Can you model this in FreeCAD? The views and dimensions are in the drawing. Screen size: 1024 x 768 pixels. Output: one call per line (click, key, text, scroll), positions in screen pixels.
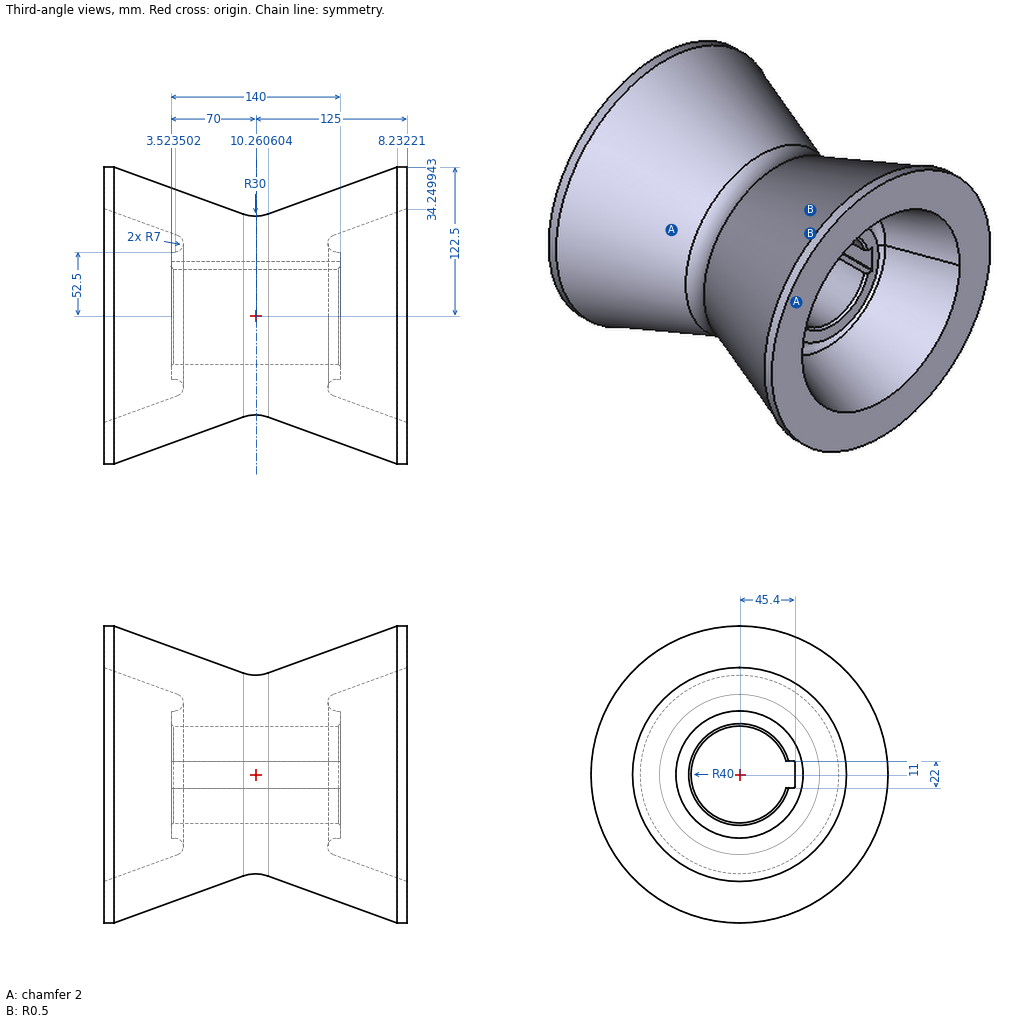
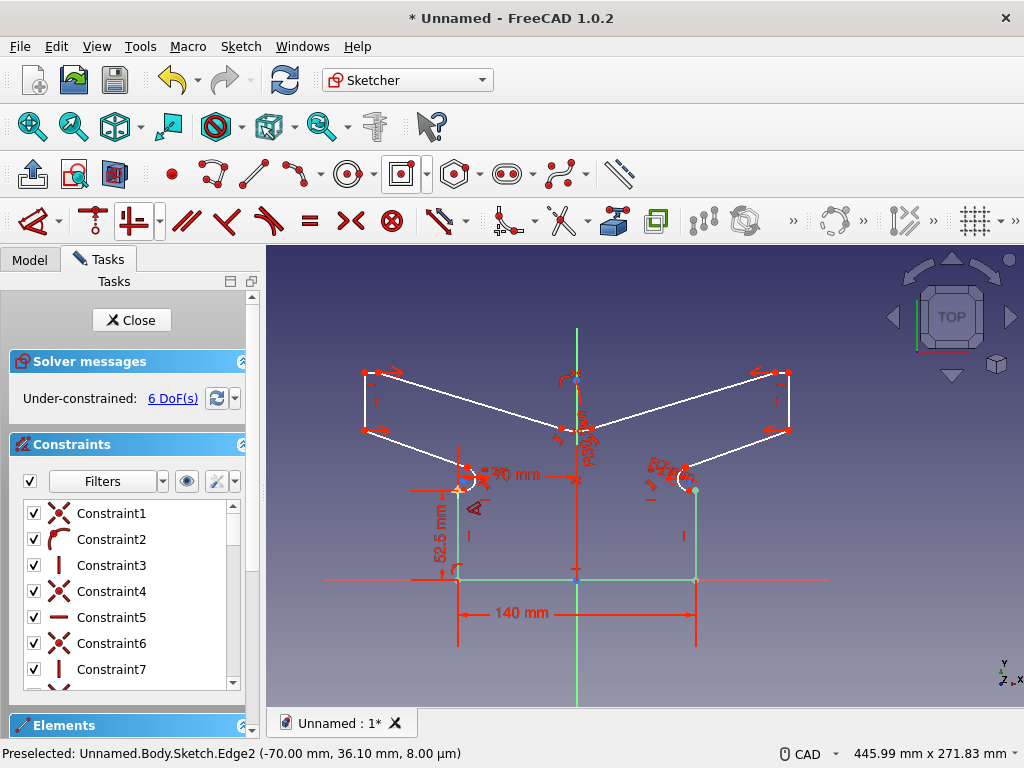
click(789, 431)
click(683, 614)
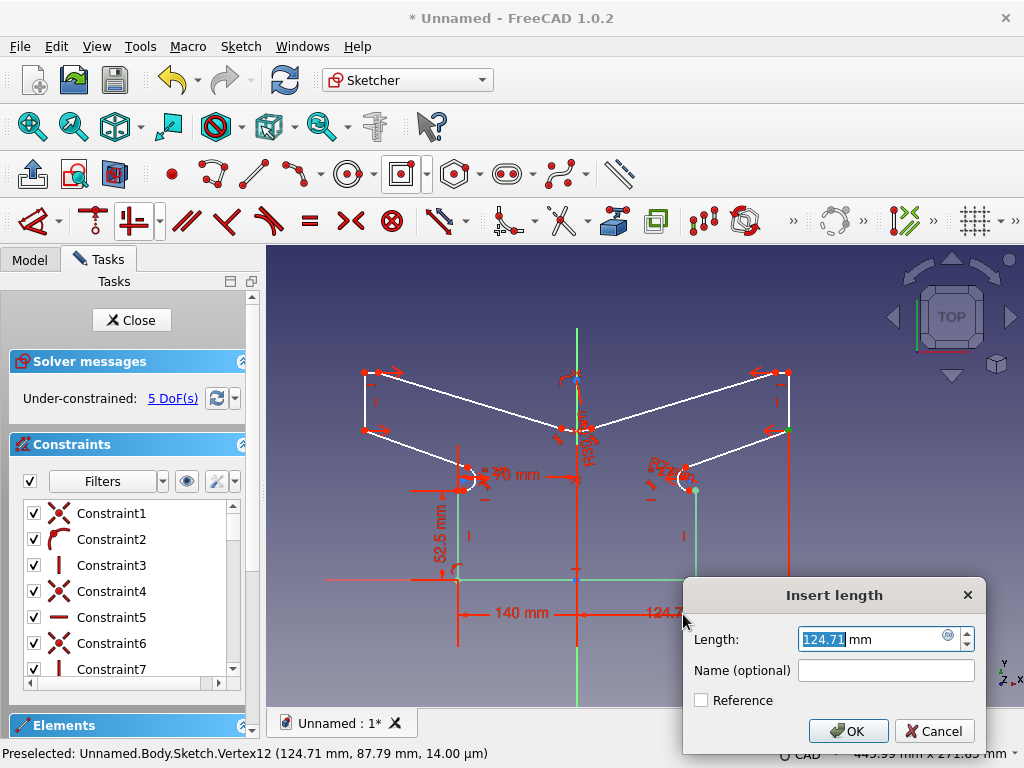
text(125)
key(Return)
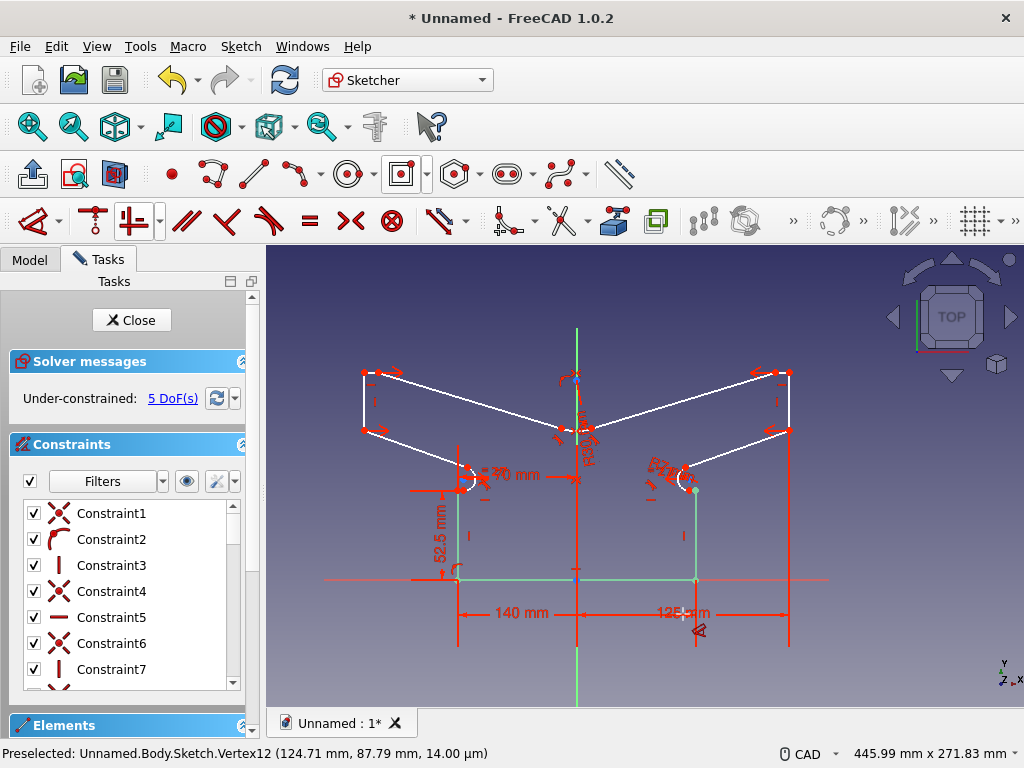
click(789, 373)
click(823, 477)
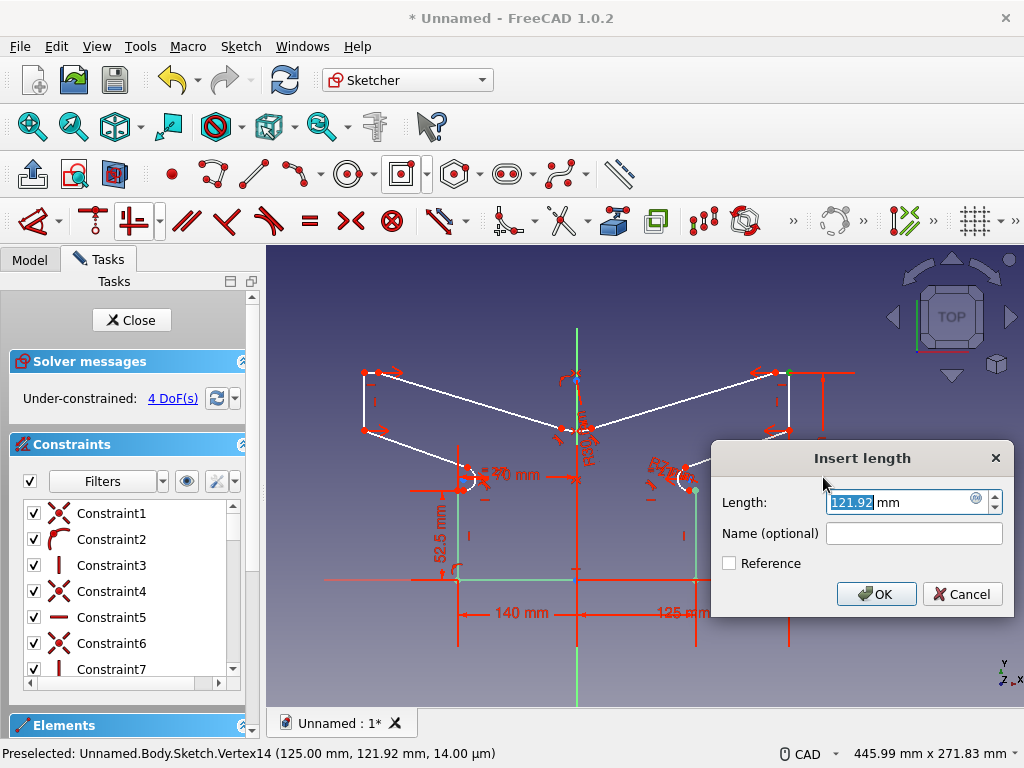
text(122.5)
key(Return)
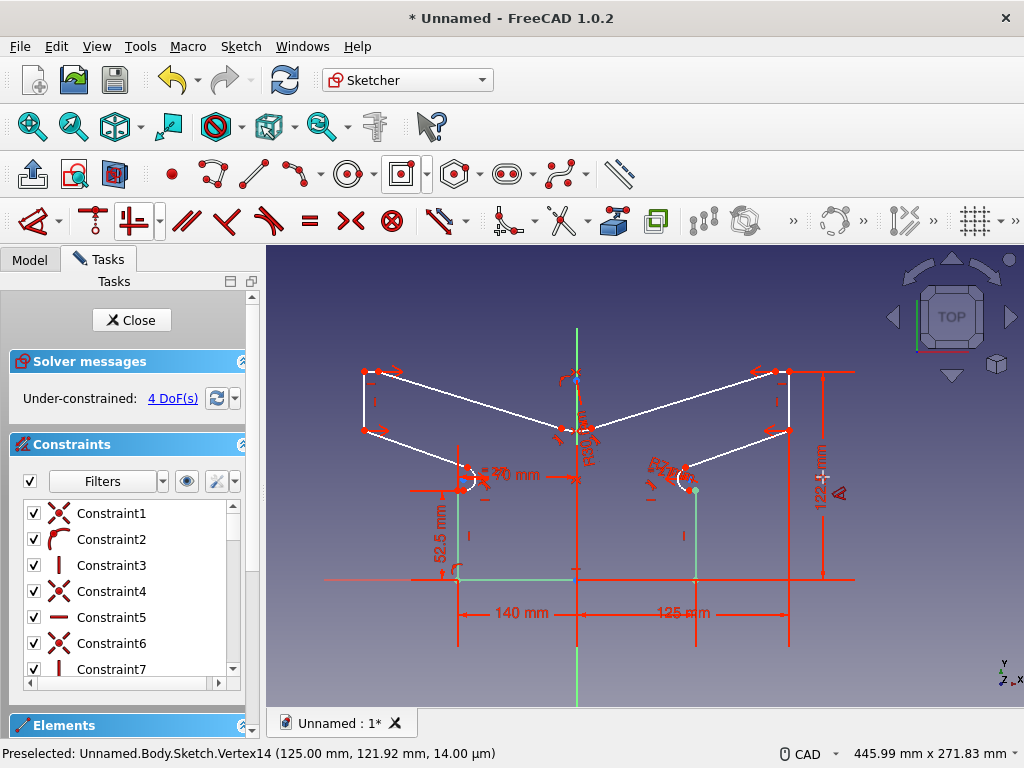
scroll(782, 372, up, 6)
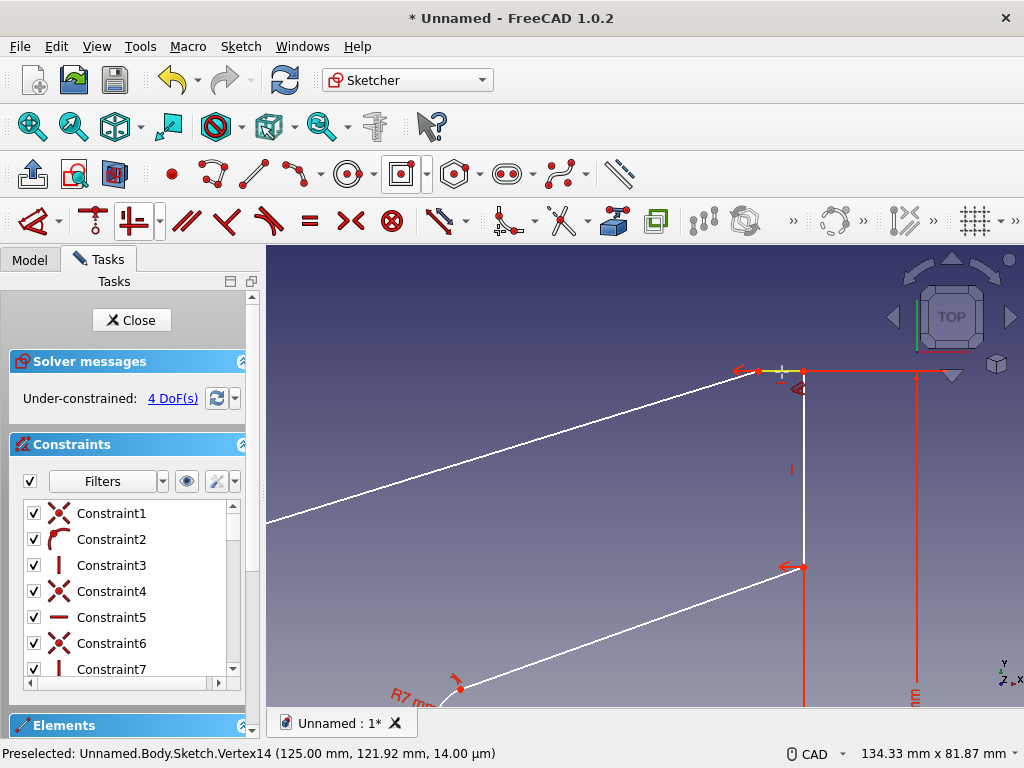
click(781, 371)
click(781, 337)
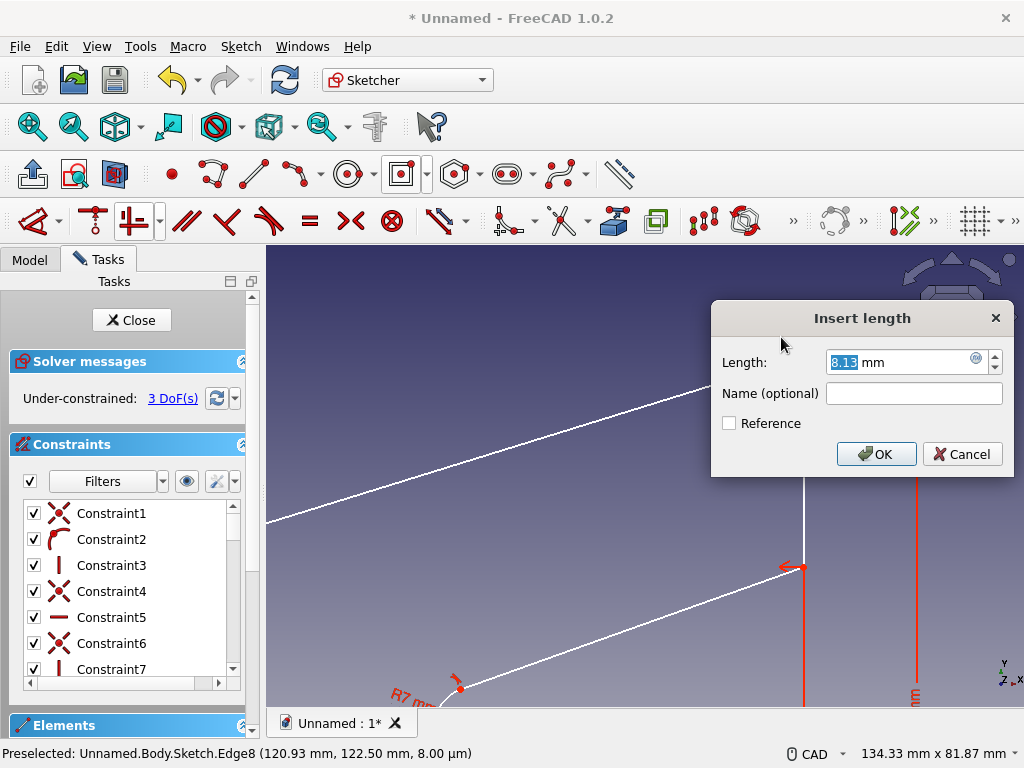
text(8.23221)
key(Return)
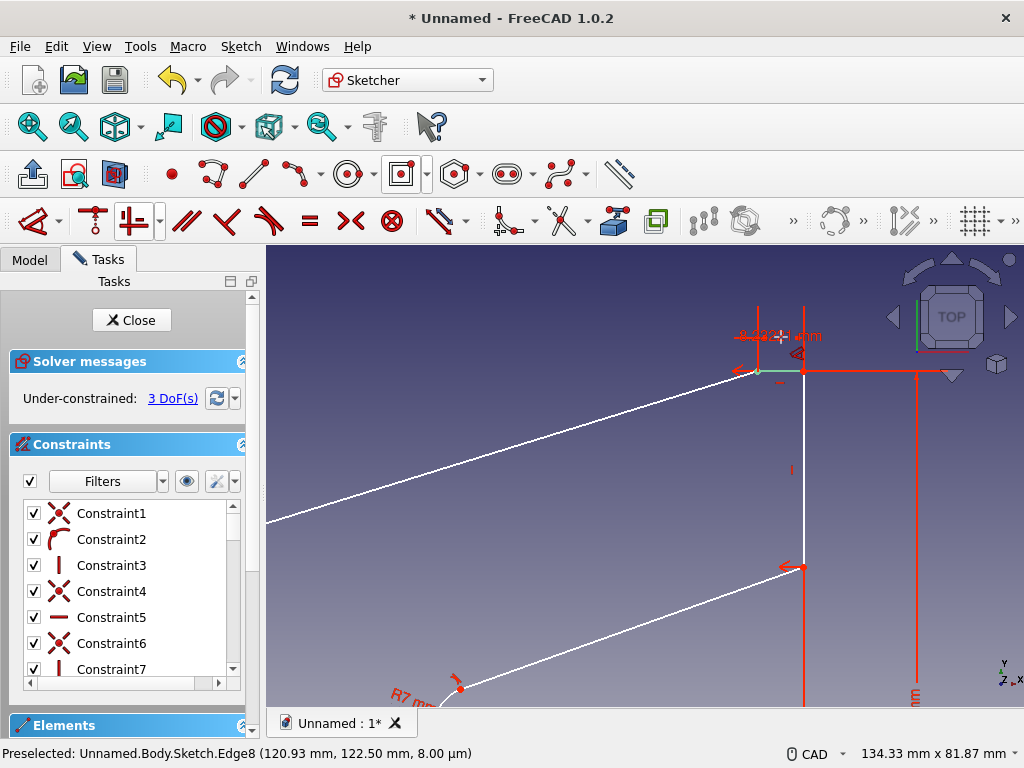
scroll(782, 372, down, 6)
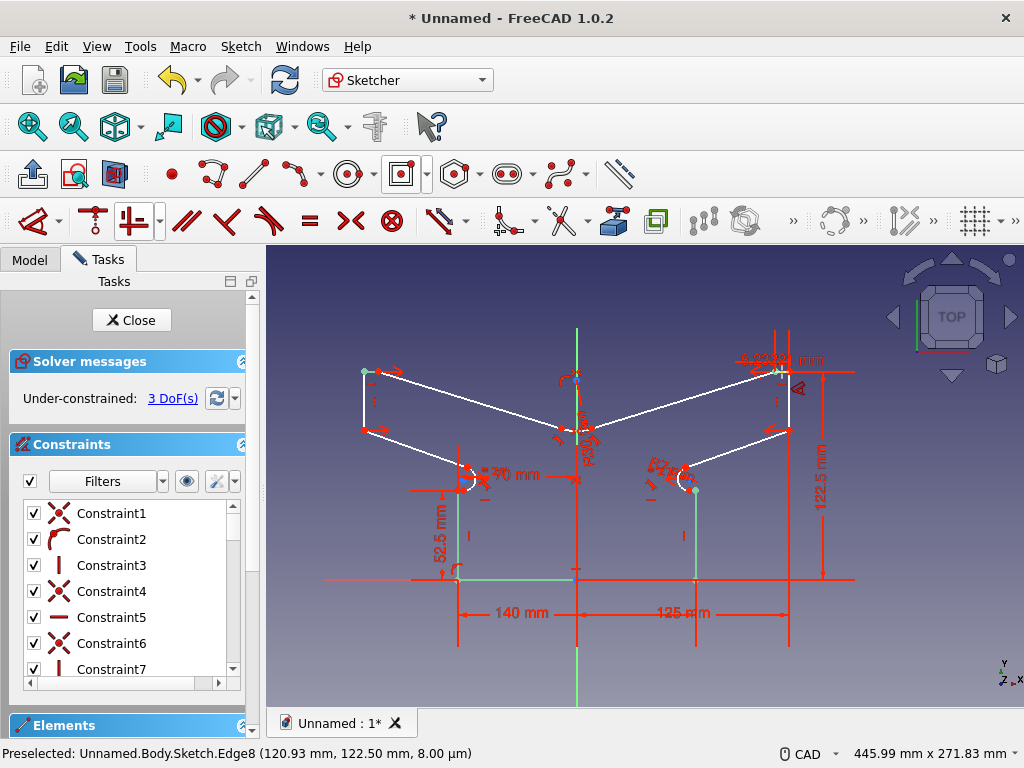
scroll(461, 491, up, 10)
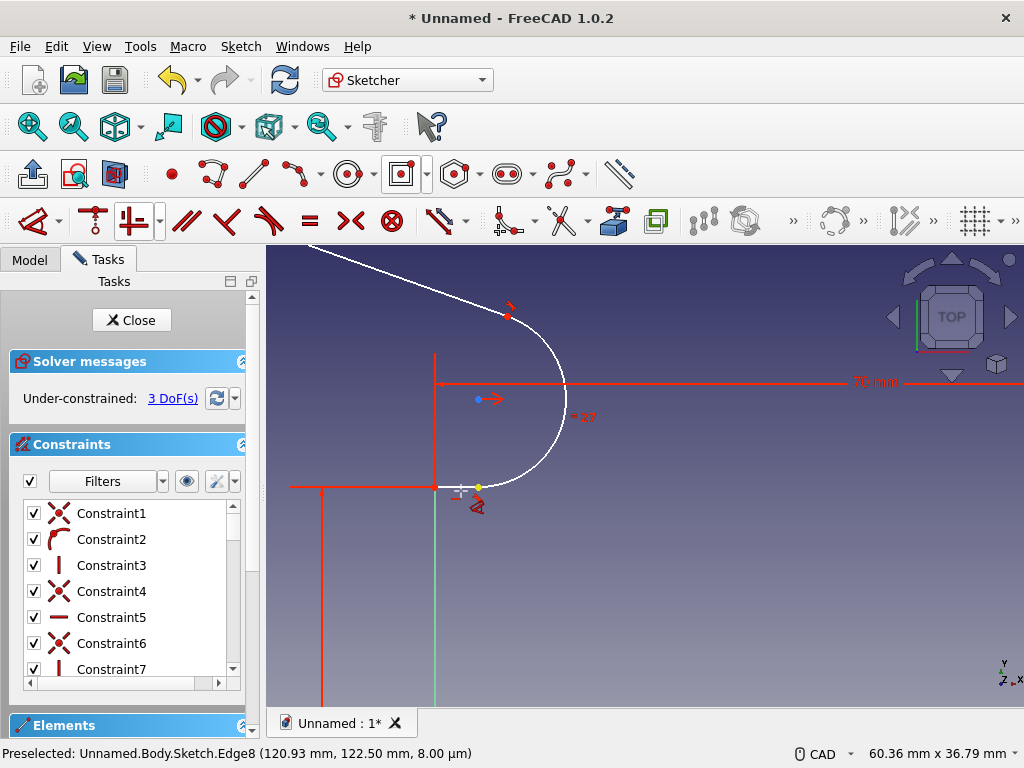
click(456, 487)
click(456, 521)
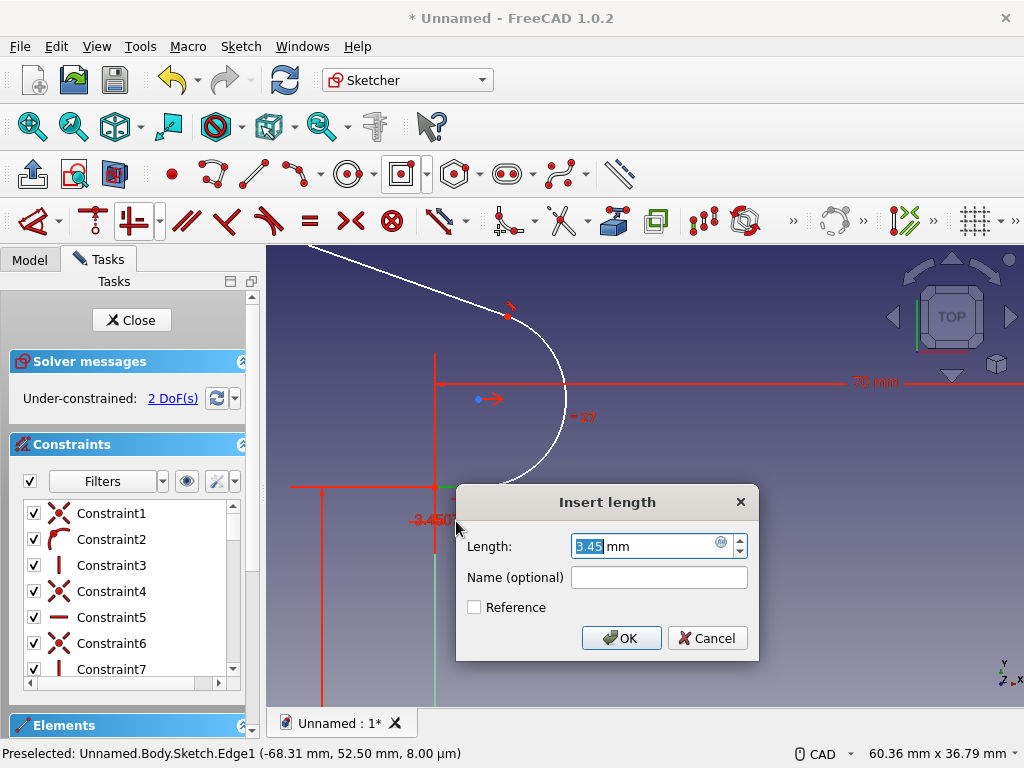
text(3.523502)
key(Return)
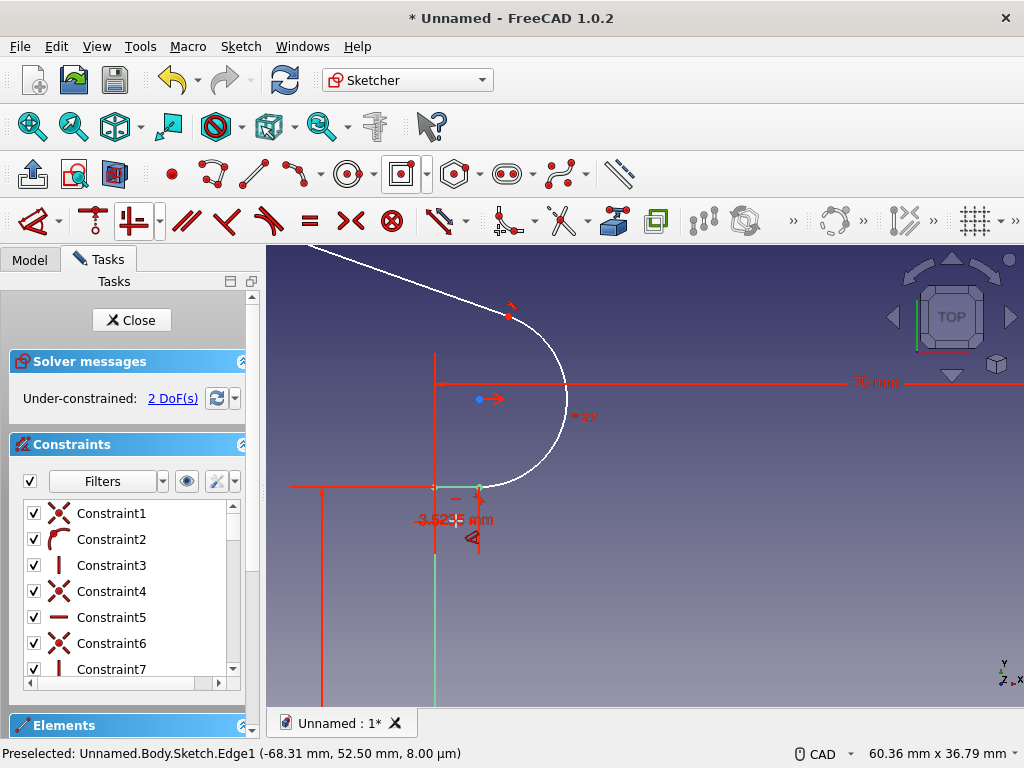
scroll(461, 491, down, 10)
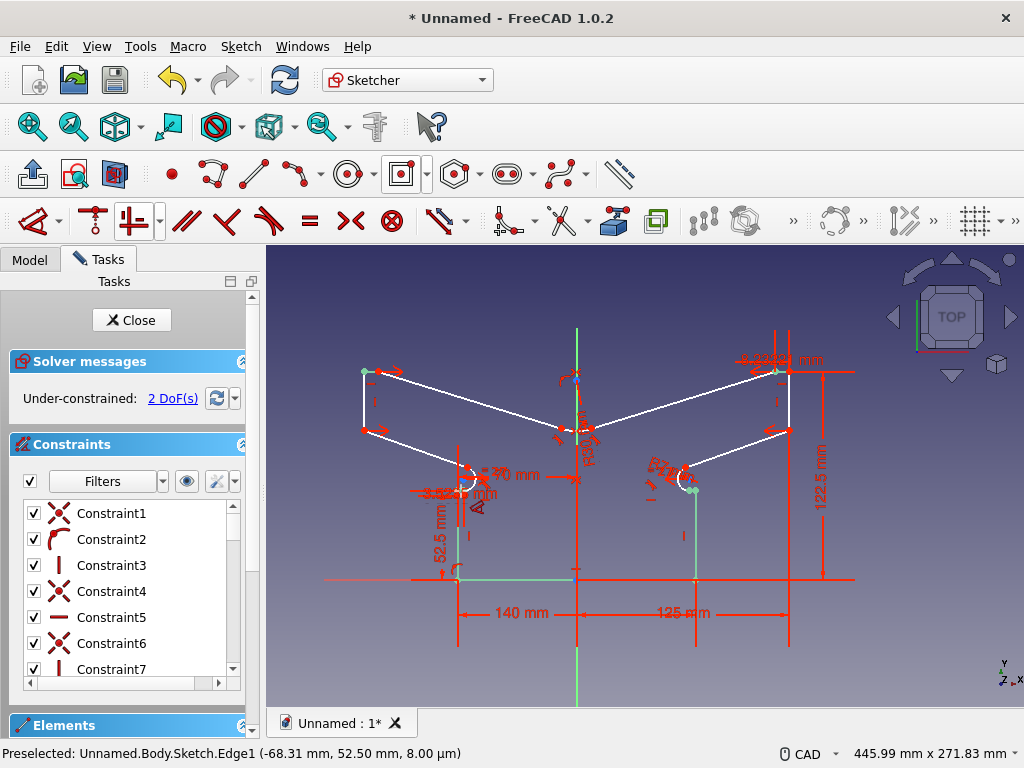
click(789, 413)
click(823, 401)